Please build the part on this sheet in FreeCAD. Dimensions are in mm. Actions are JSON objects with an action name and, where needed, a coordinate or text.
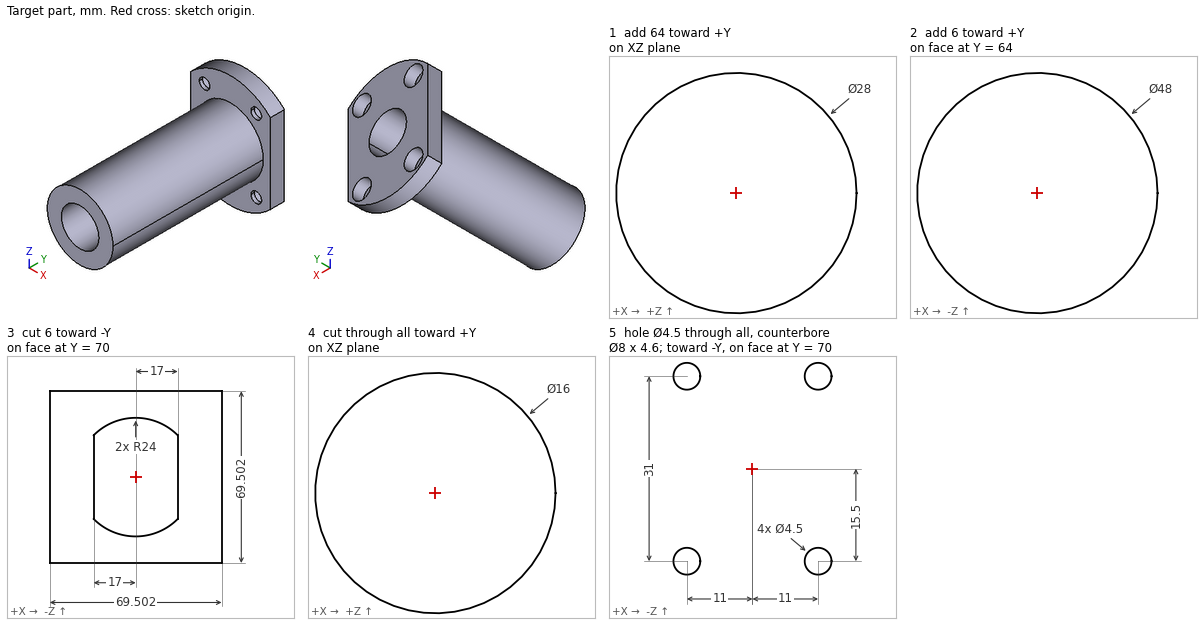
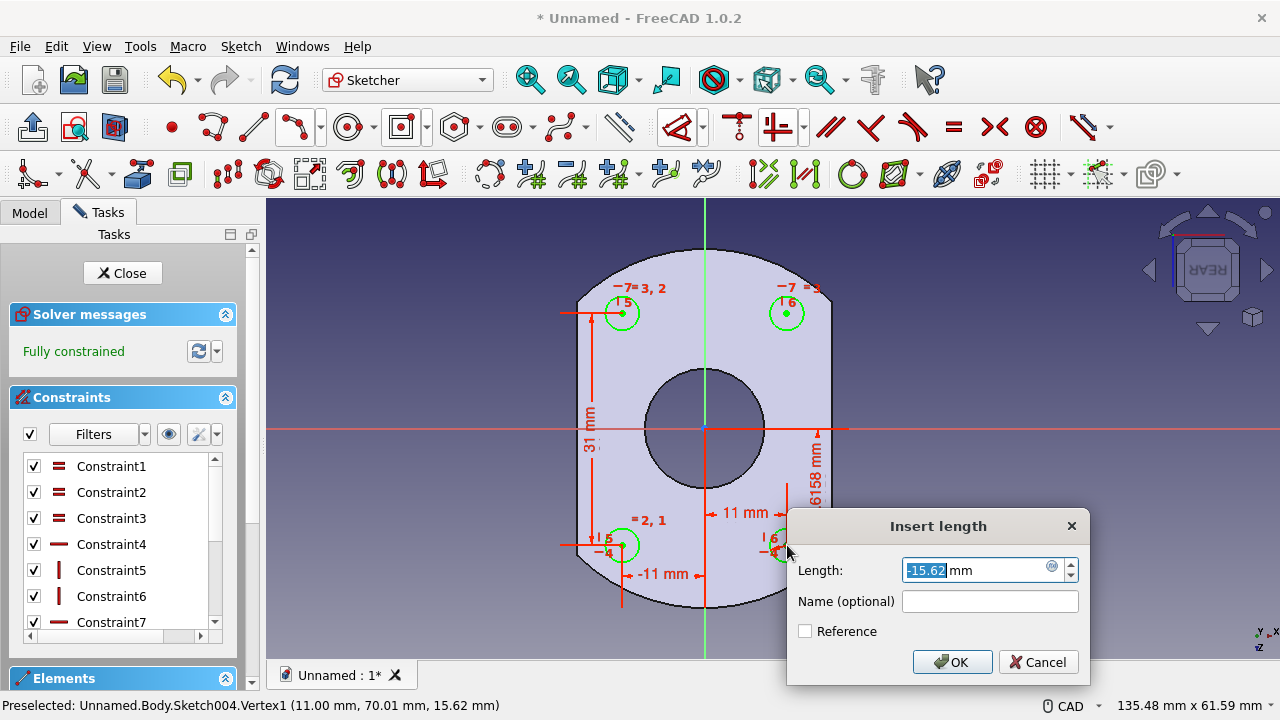
{"action": "type", "text": "-15.5"}
{"action": "key", "text": "Return"}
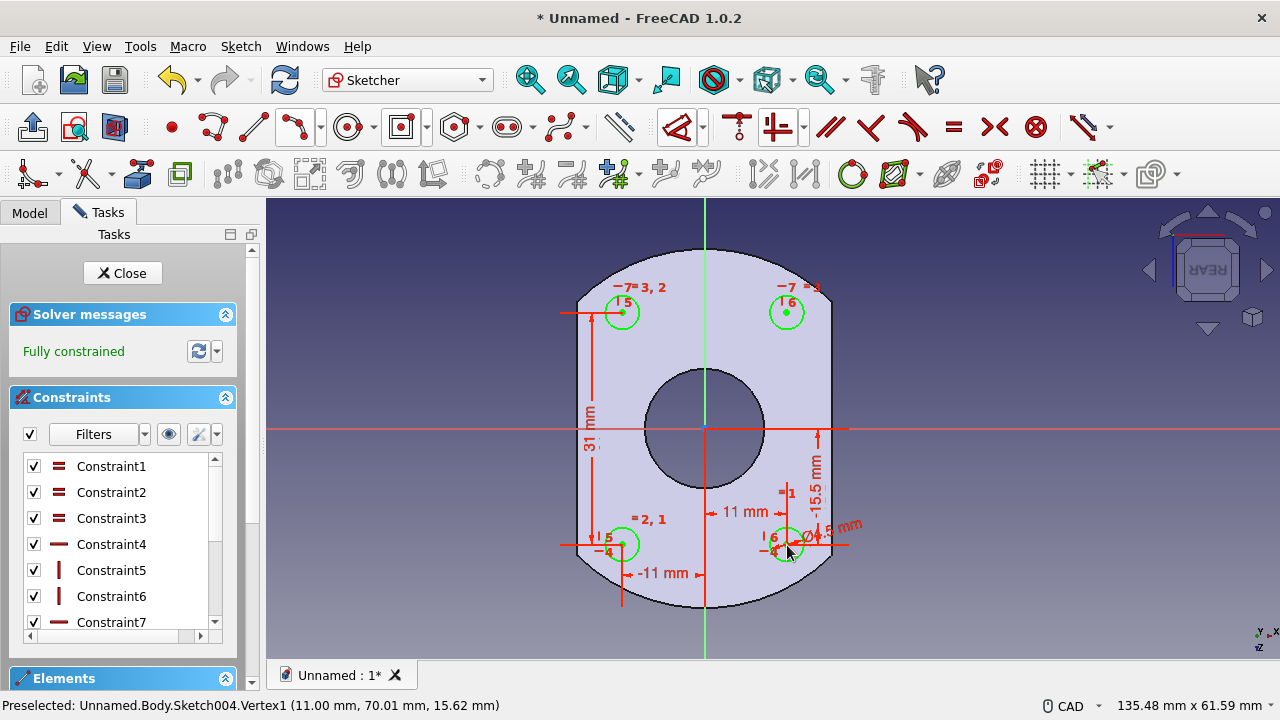
{"action": "left_click", "coordinate": [123, 273]}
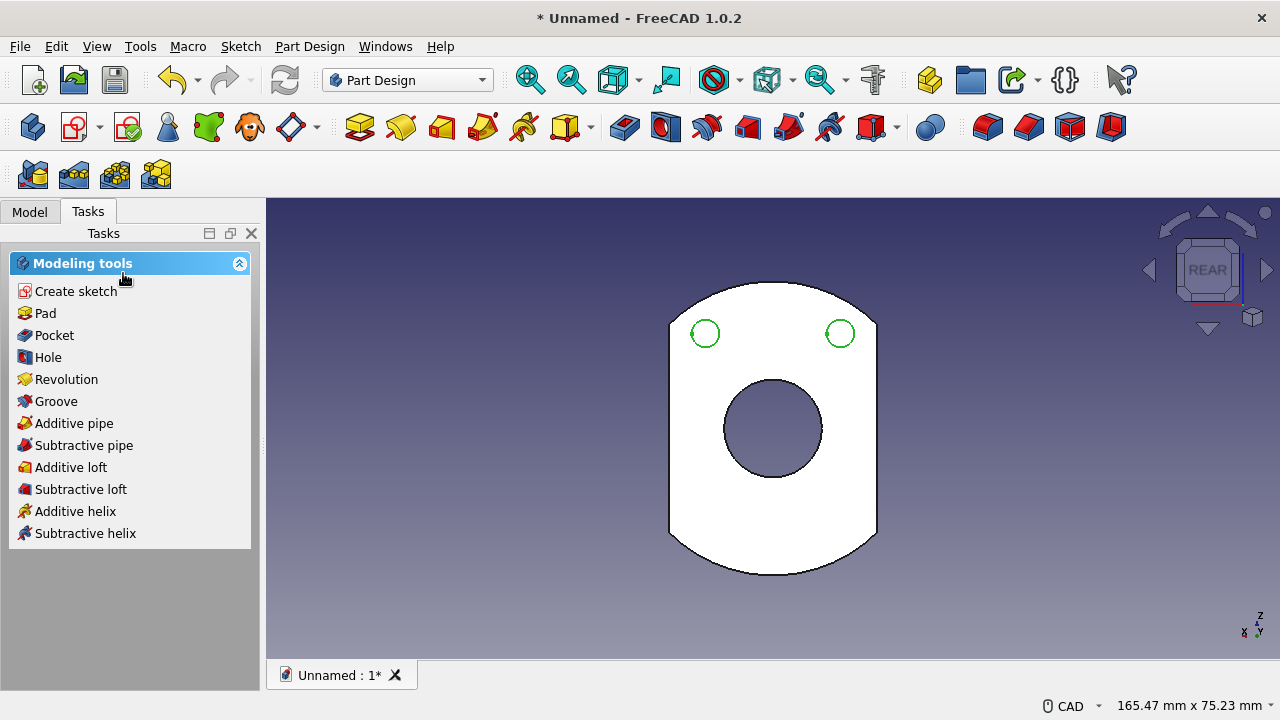
{"action": "left_click", "coordinate": [666, 128]}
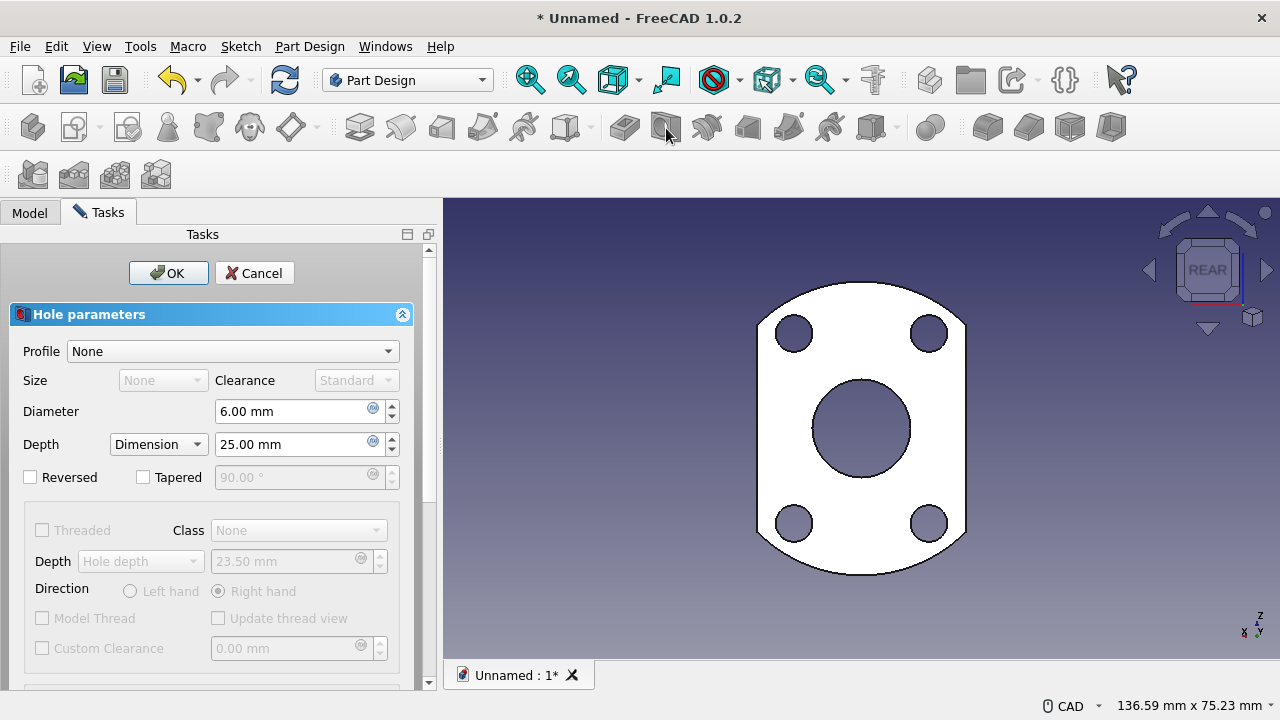
{"action": "triple_click", "coordinate": [300, 412]}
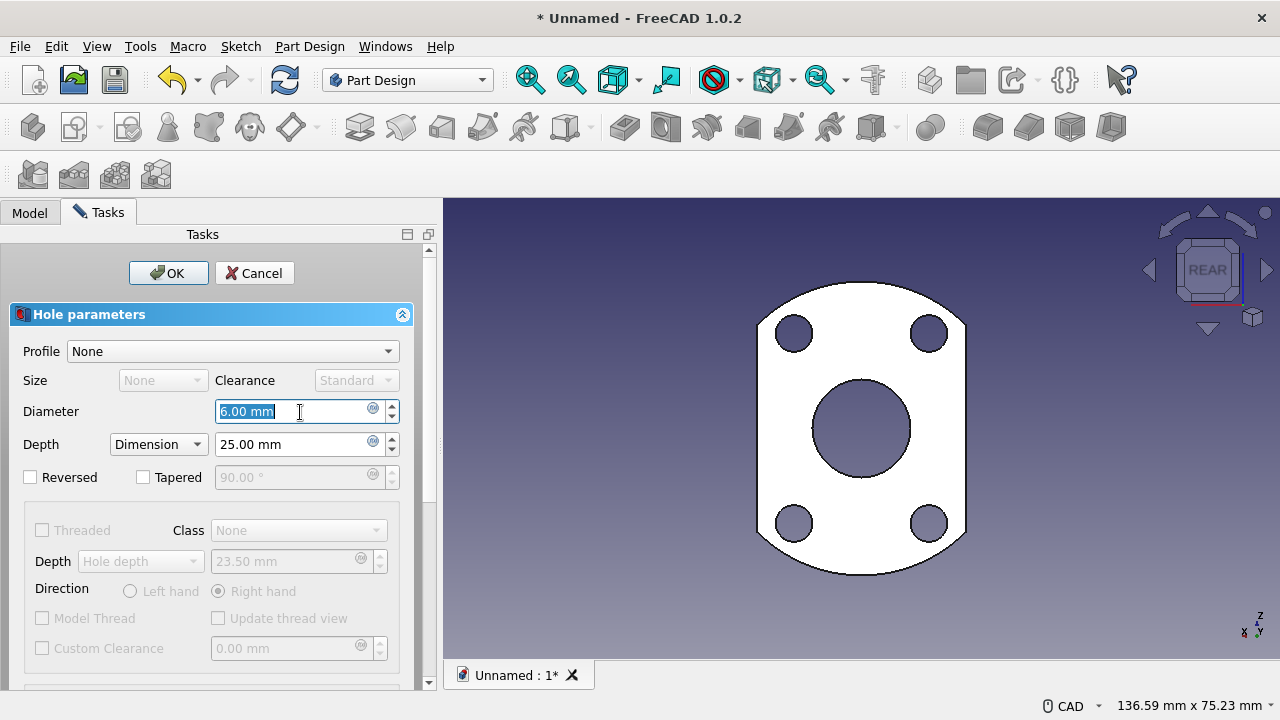
{"action": "type", "text": "4.5"}
{"action": "key", "text": "Tab"}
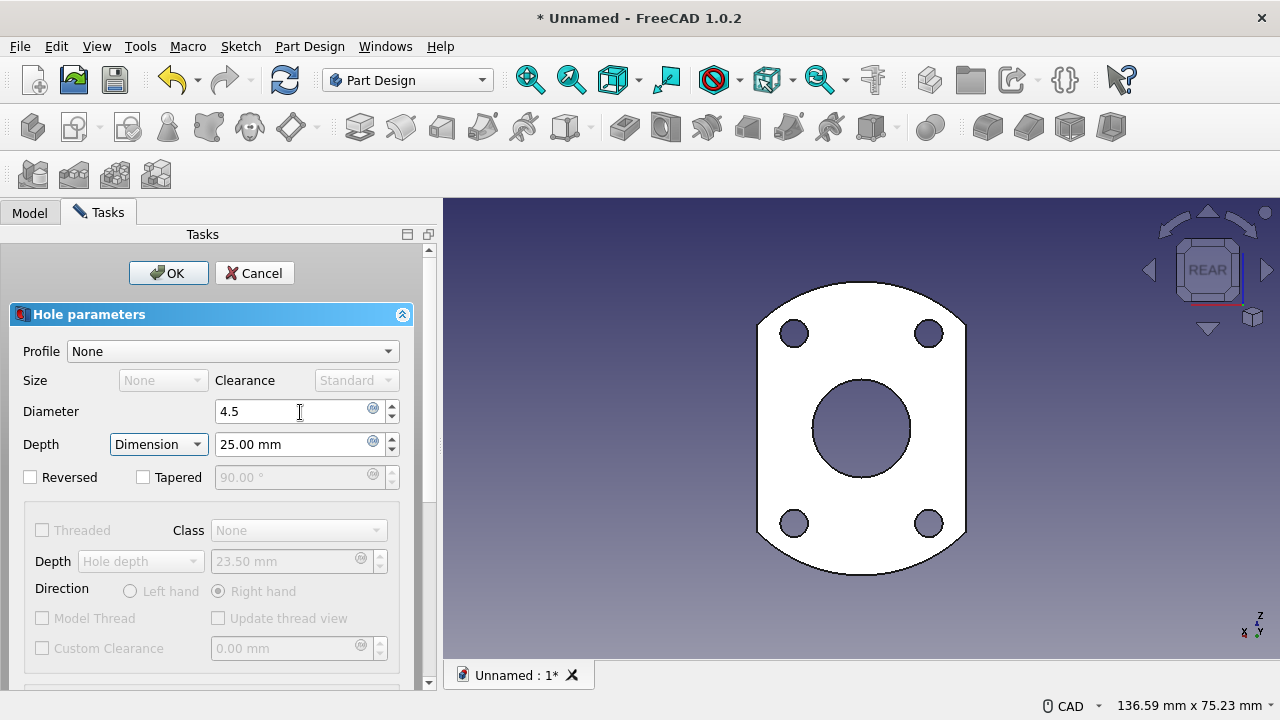
{"action": "left_click", "coordinate": [160, 444]}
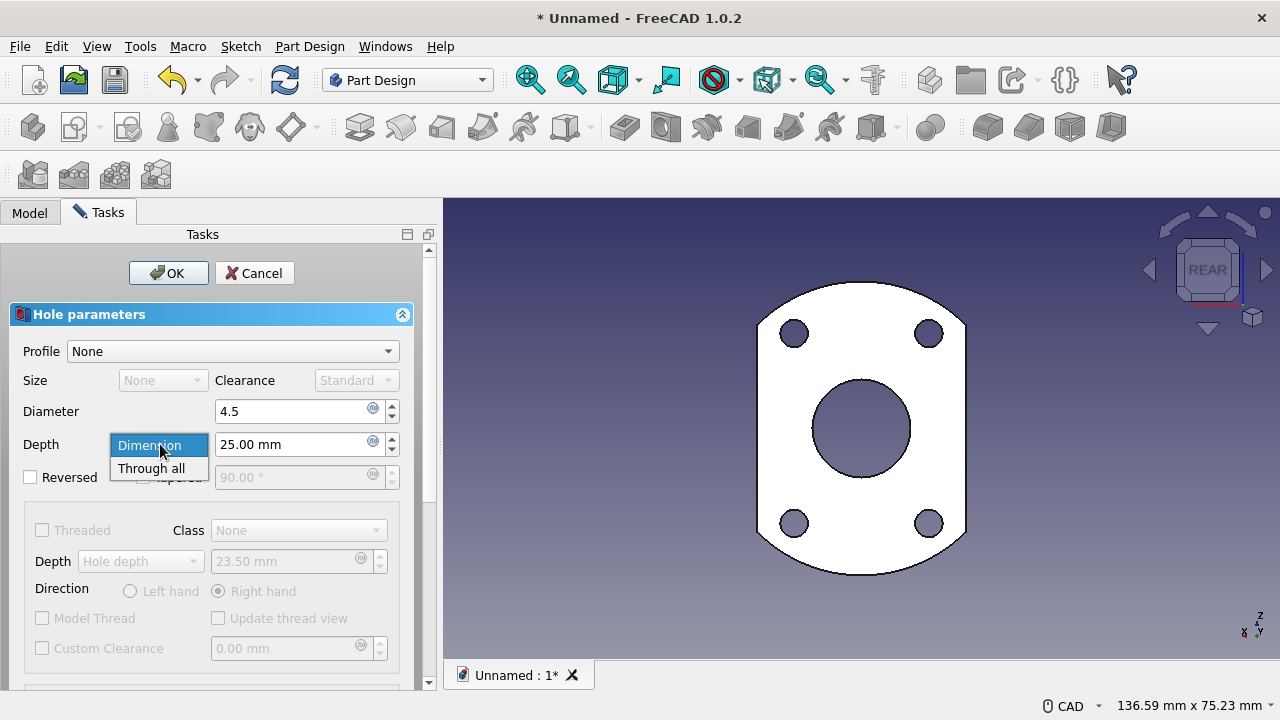
{"action": "left_click", "coordinate": [158, 468]}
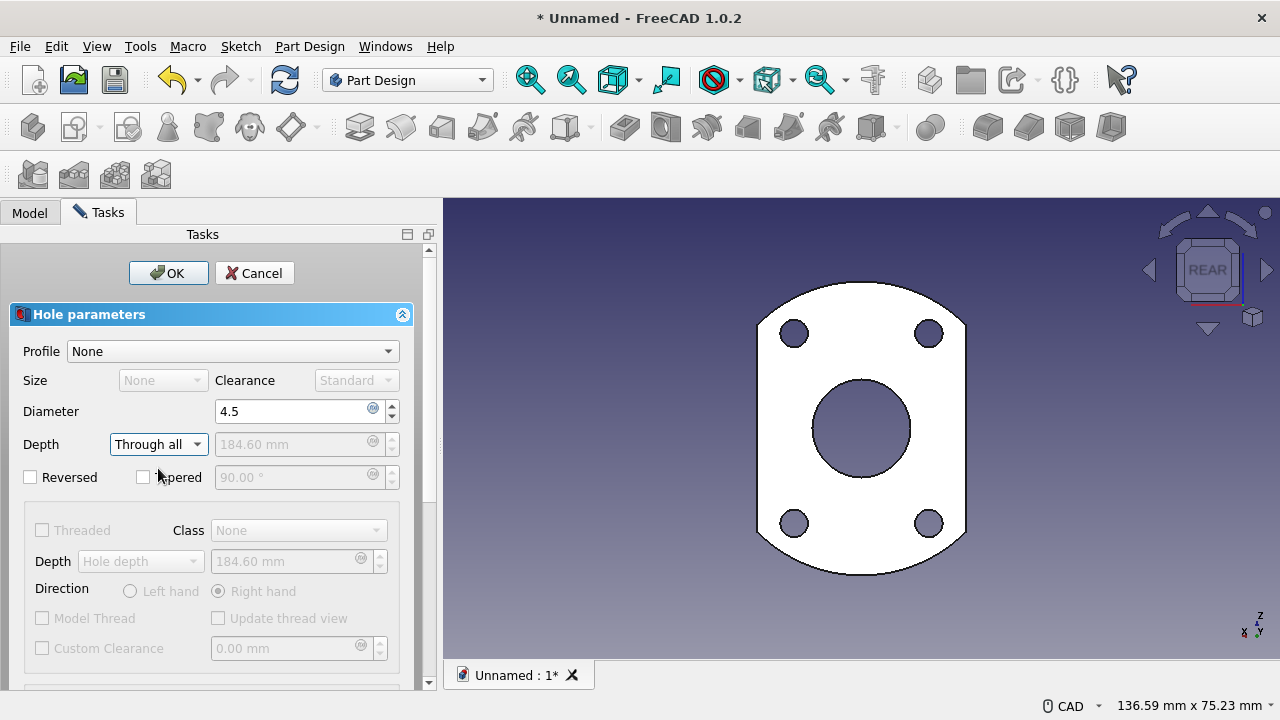
{"action": "scroll", "coordinate": [429, 467], "scroll_direction": "down", "scroll_amount": 2}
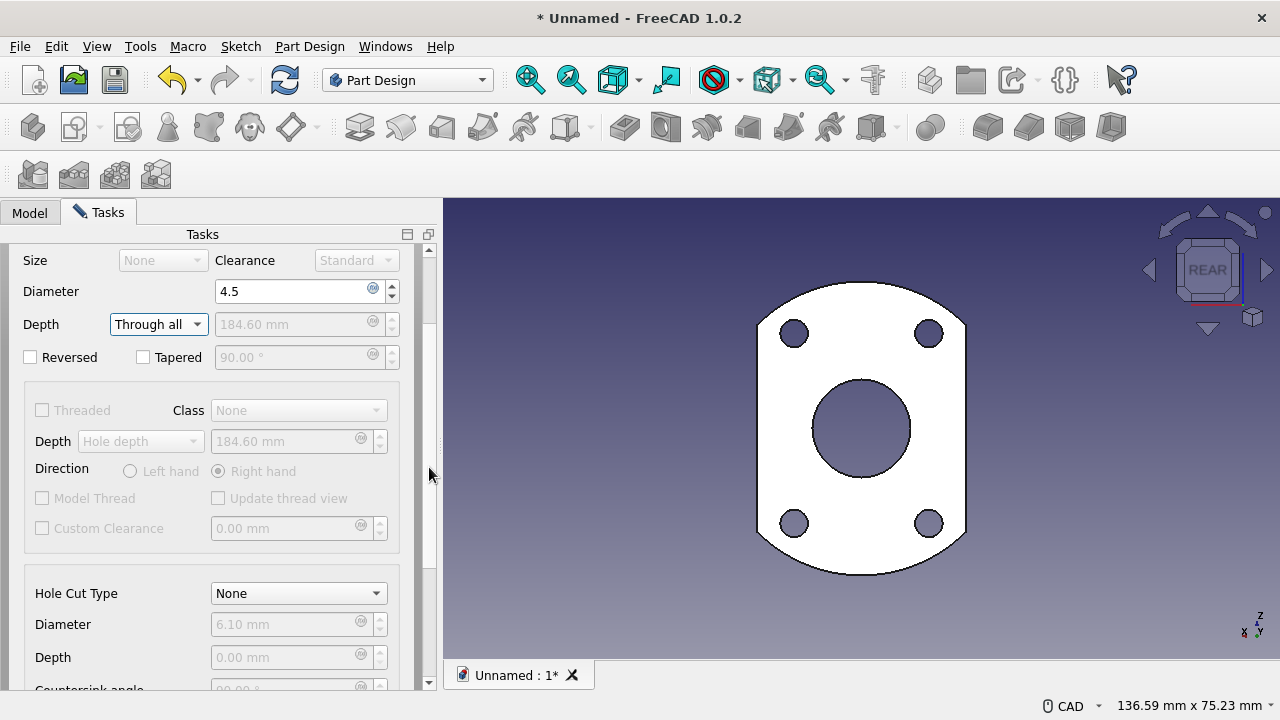
{"action": "left_click", "coordinate": [300, 594]}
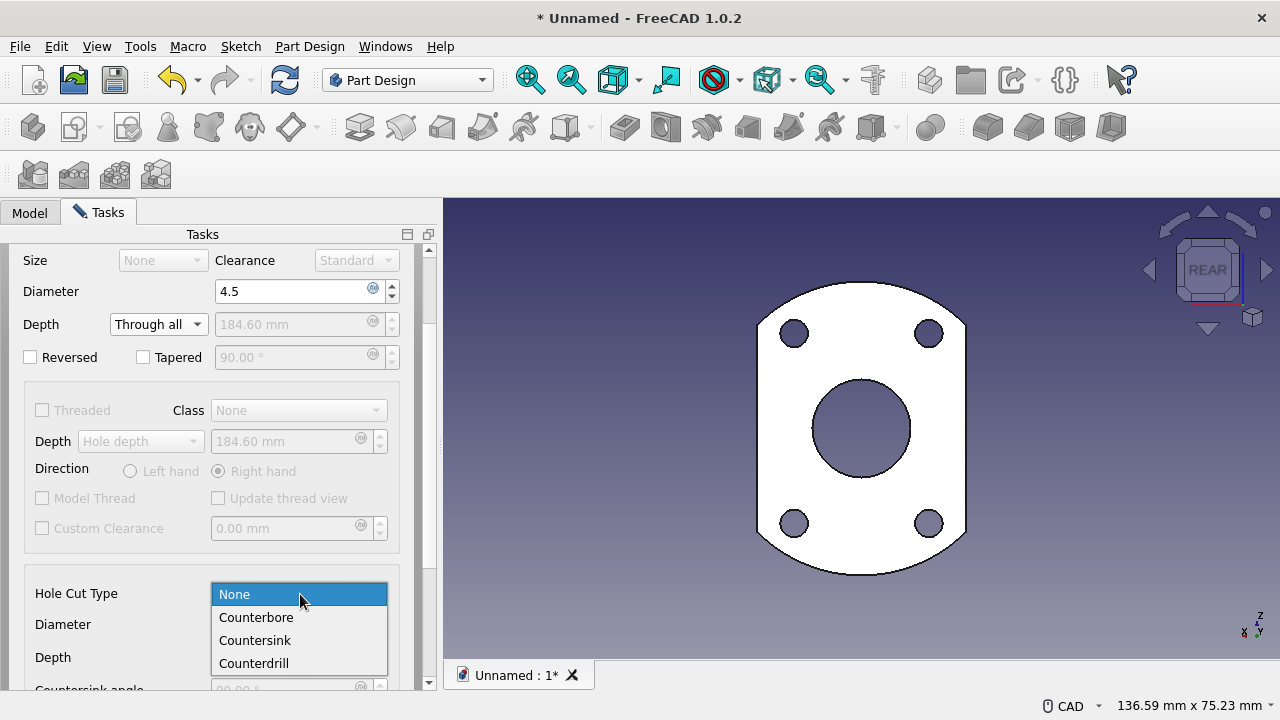
{"action": "left_click", "coordinate": [298, 618]}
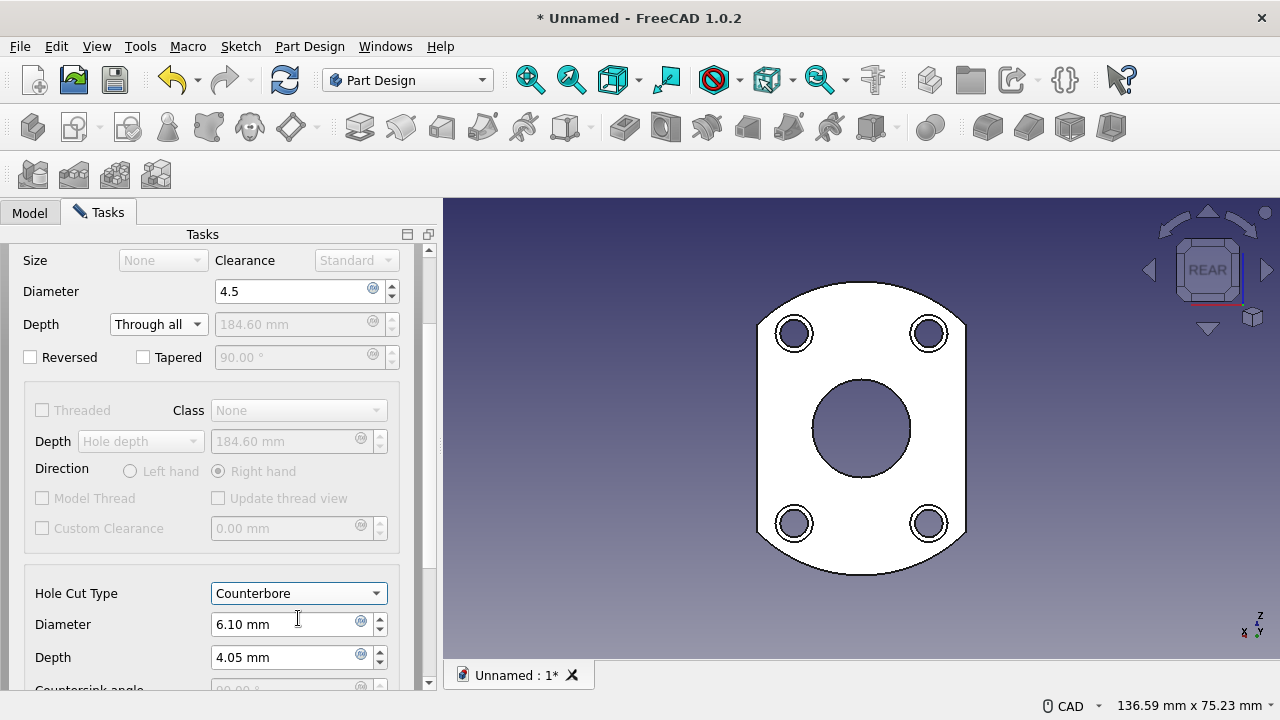
{"action": "triple_click", "coordinate": [292, 624]}